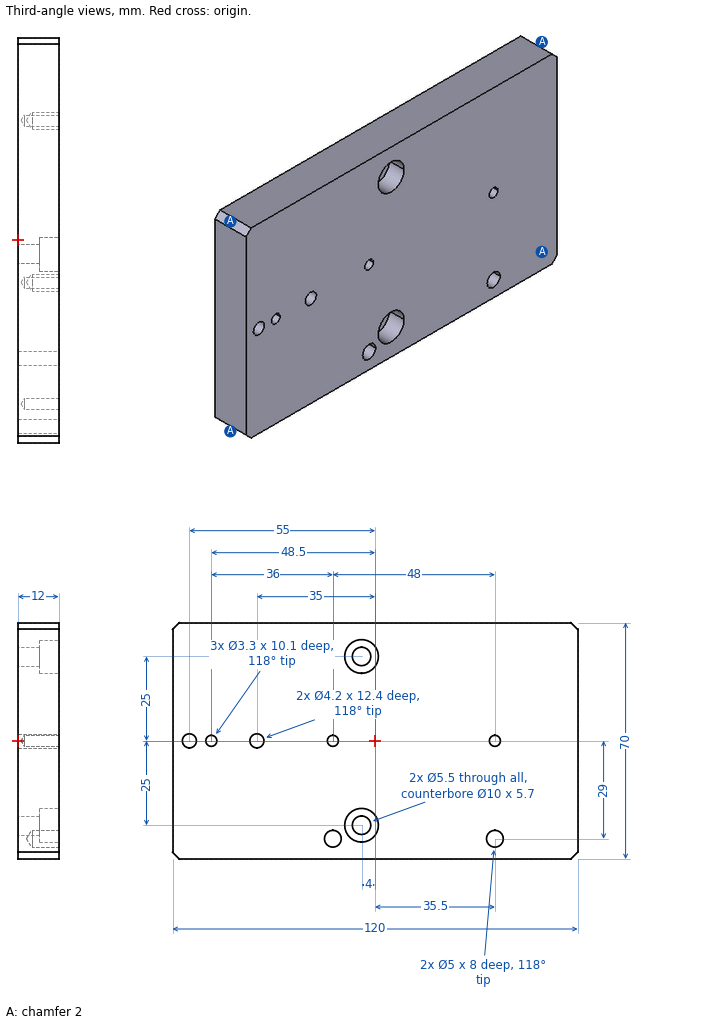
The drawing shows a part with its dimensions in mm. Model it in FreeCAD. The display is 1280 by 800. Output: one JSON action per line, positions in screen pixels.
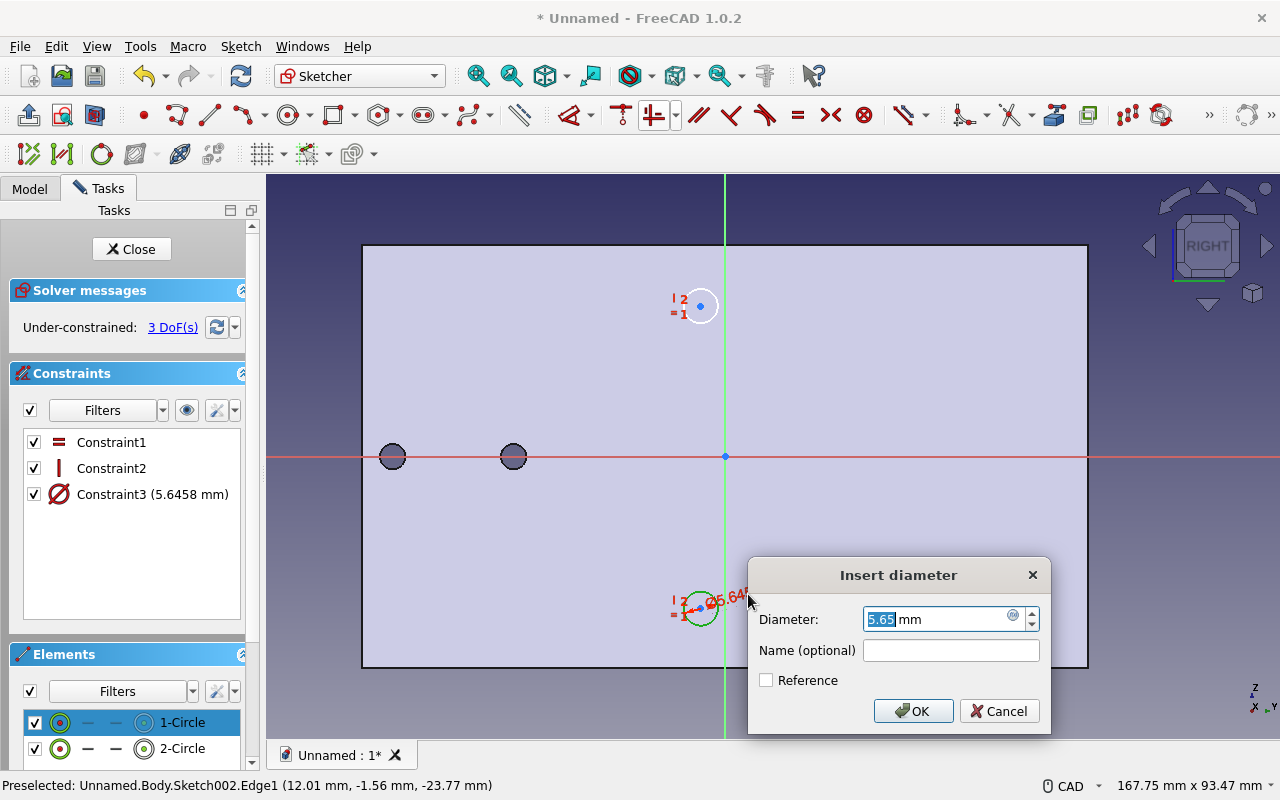
{"action": "type", "text": "5.5"}
{"action": "key", "text": "Return"}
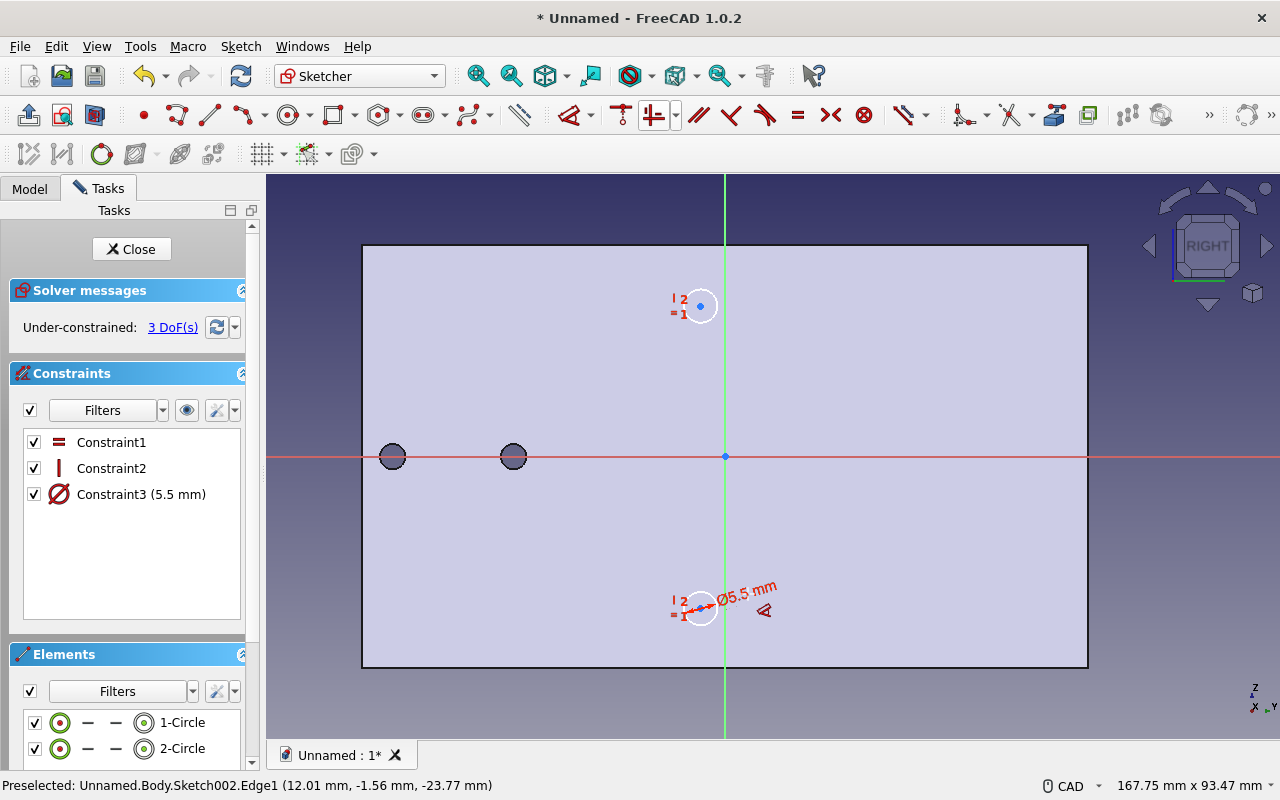
{"action": "scroll", "coordinate": [701, 609], "scroll_direction": "up", "scroll_amount": 3}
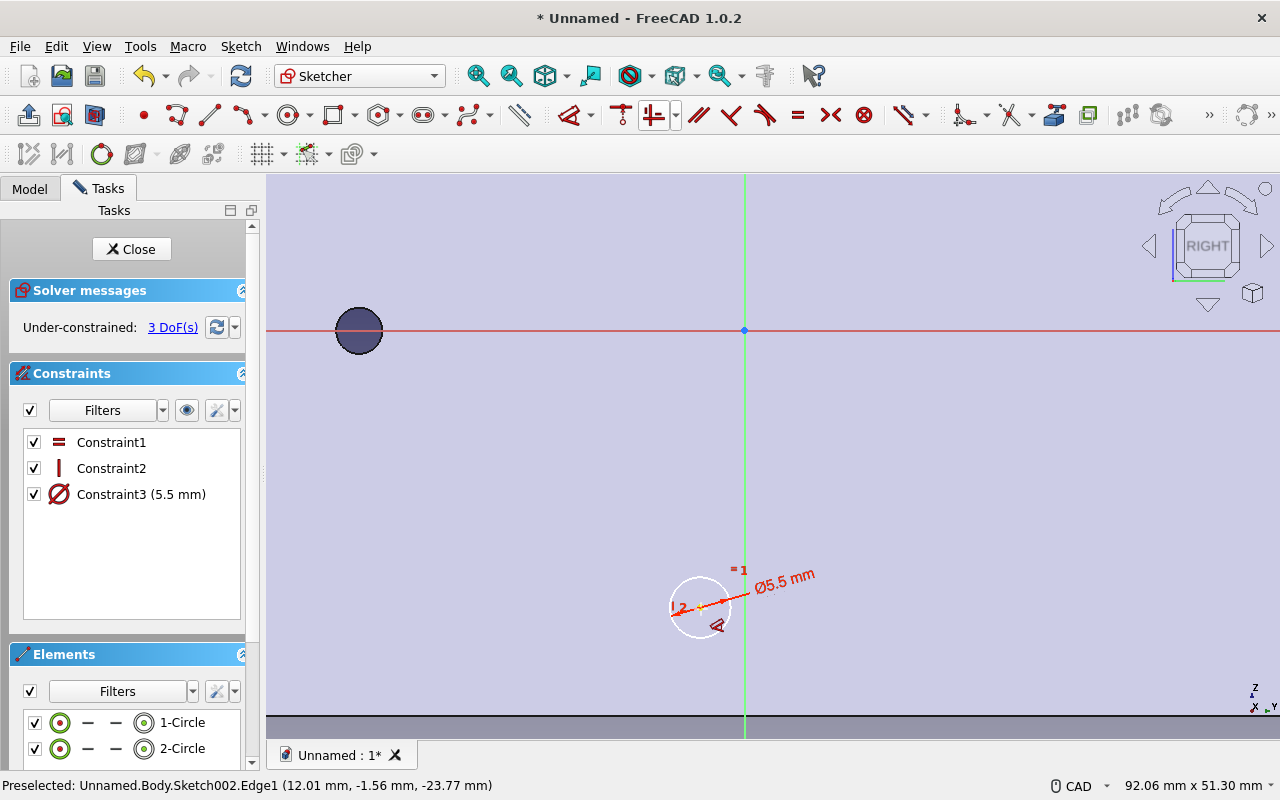
{"action": "left_click", "coordinate": [700, 608]}
{"action": "left_click", "coordinate": [722, 297]}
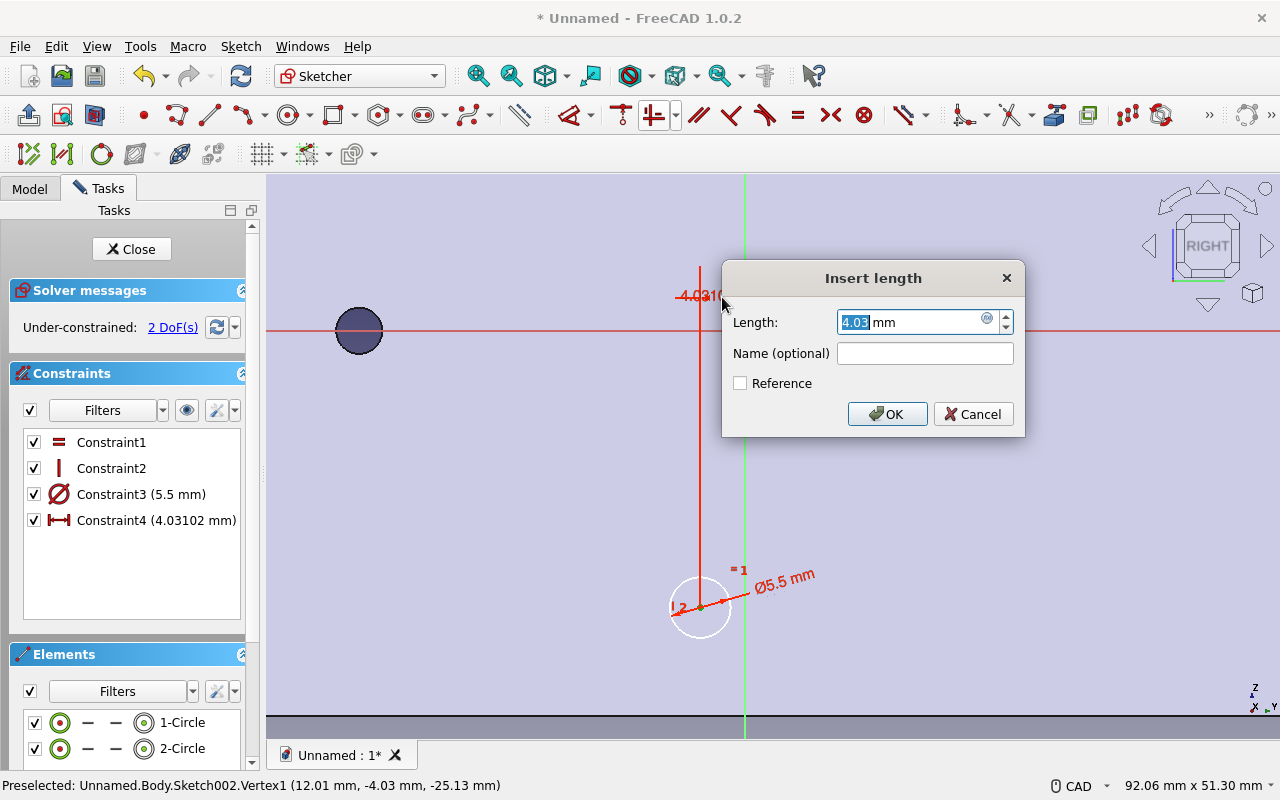
{"action": "type", "text": "4"}
{"action": "key", "text": "Return"}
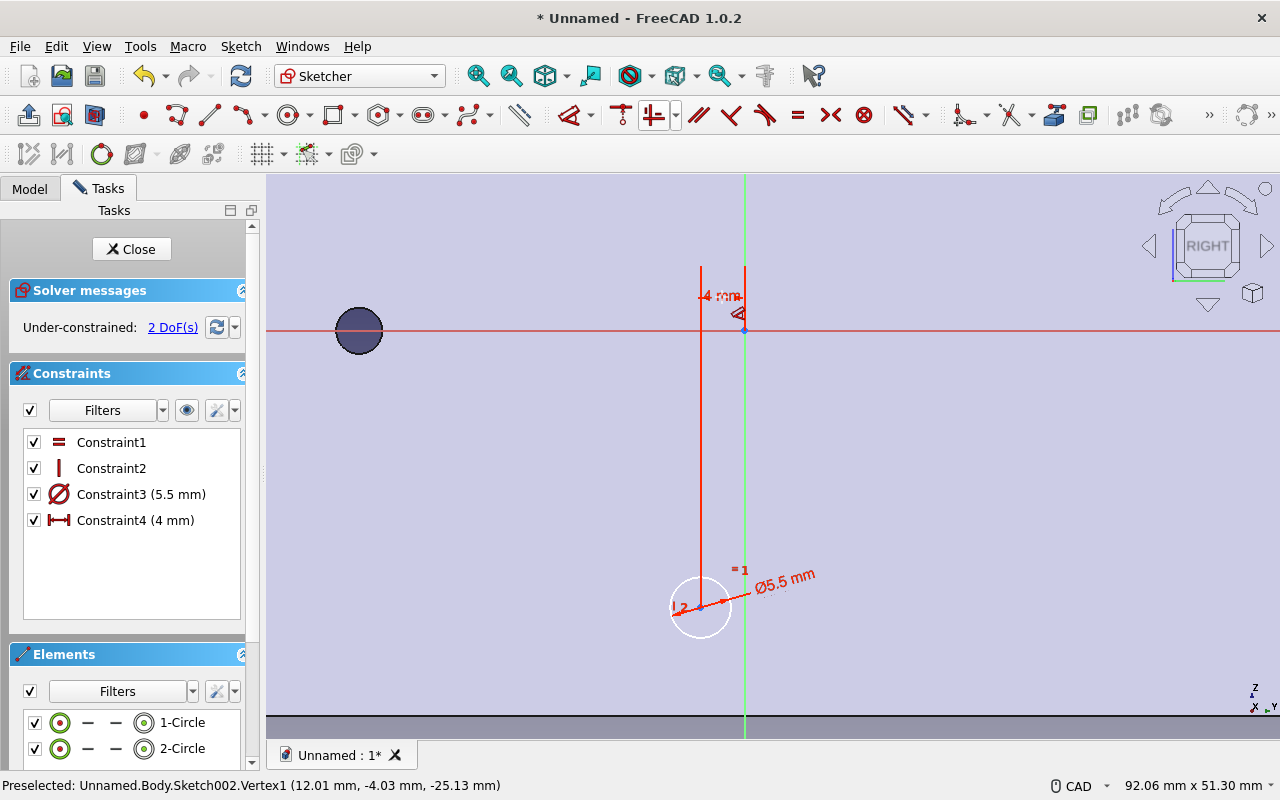
{"action": "left_click", "coordinate": [701, 608]}
{"action": "left_click", "coordinate": [779, 469]}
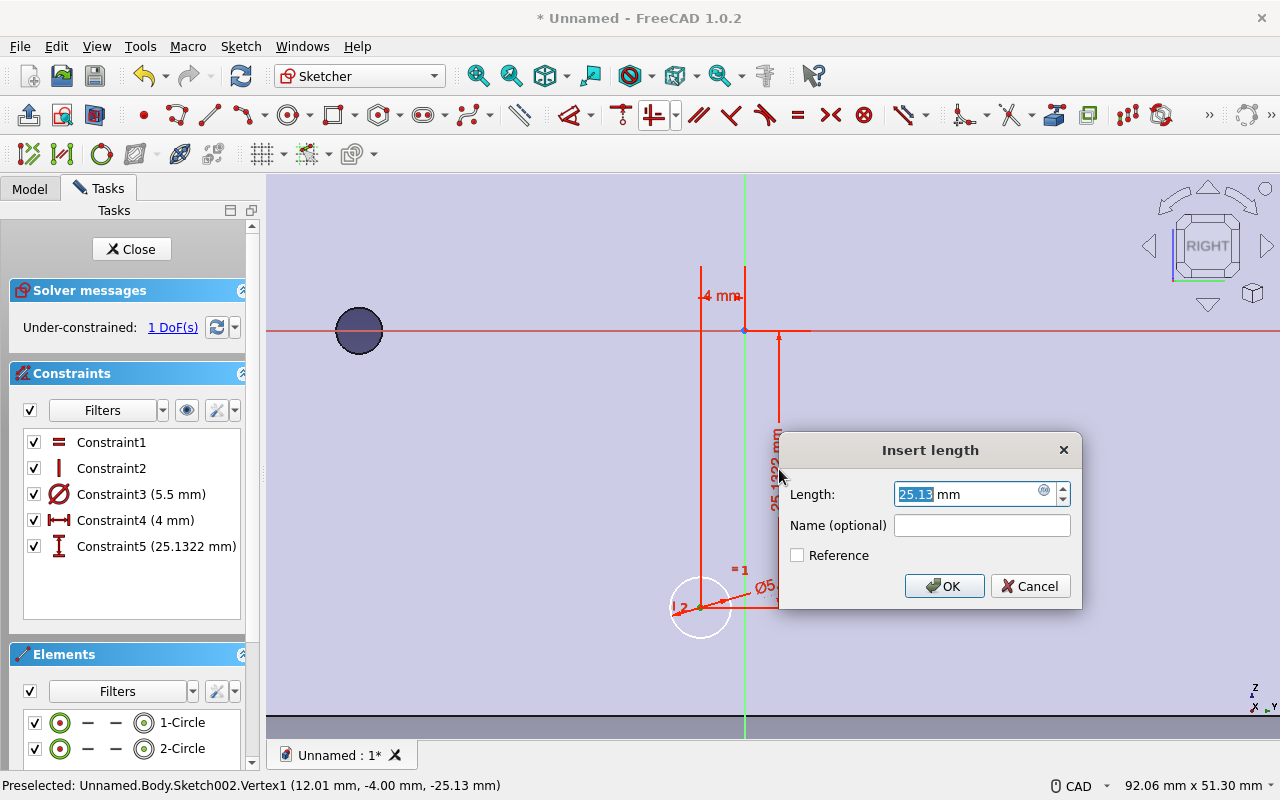
{"action": "type", "text": "25"}
{"action": "key", "text": "Return"}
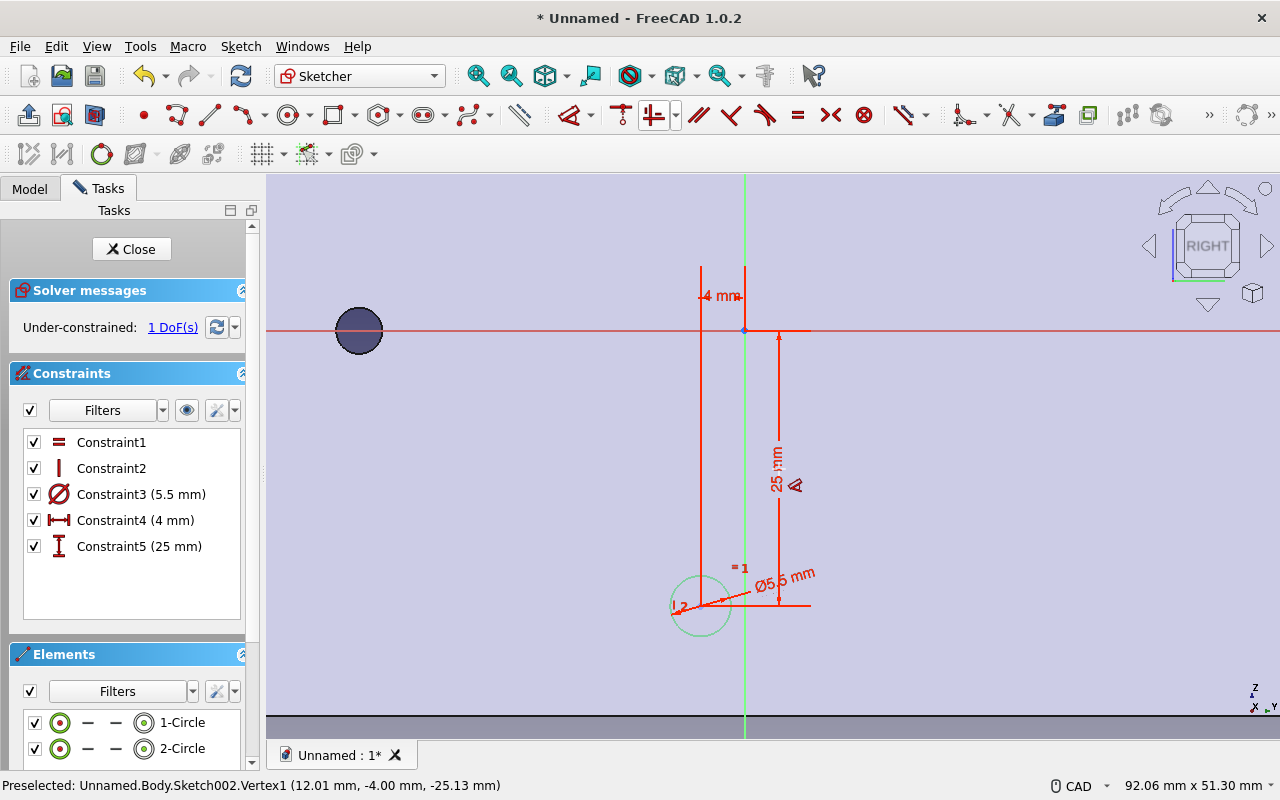
{"action": "scroll", "coordinate": [701, 609], "scroll_direction": "down", "scroll_amount": 3}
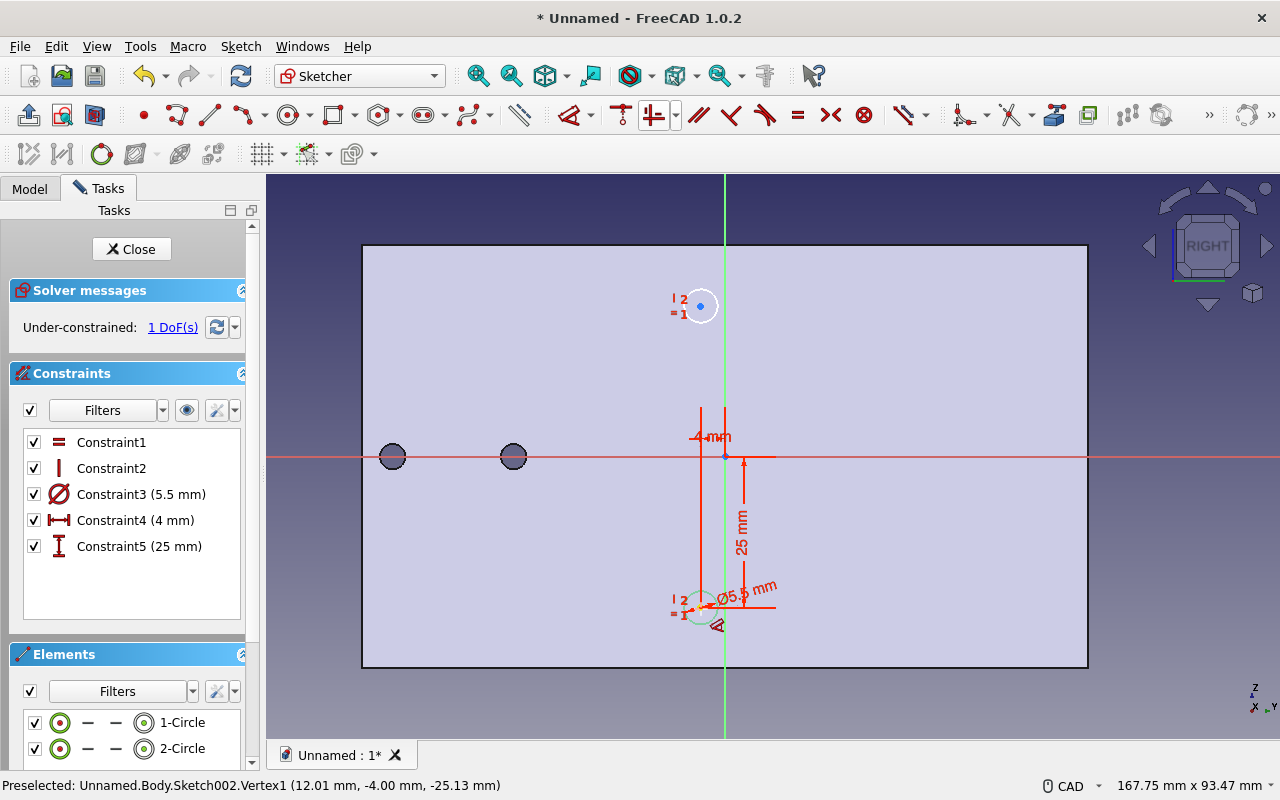
{"action": "left_click", "coordinate": [701, 306]}
{"action": "left_click", "coordinate": [759, 381]}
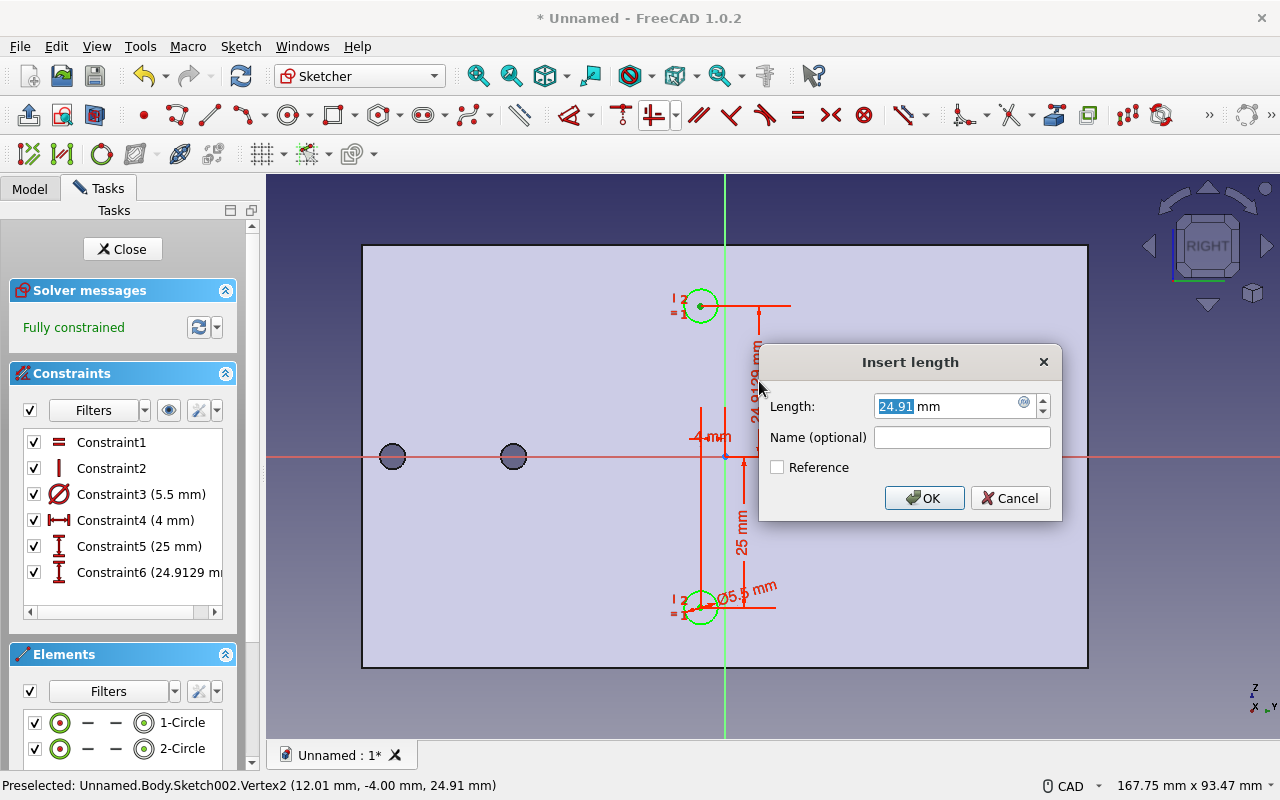
{"action": "type", "text": "25"}
{"action": "key", "text": "Return"}
{"action": "key", "text": "Escape"}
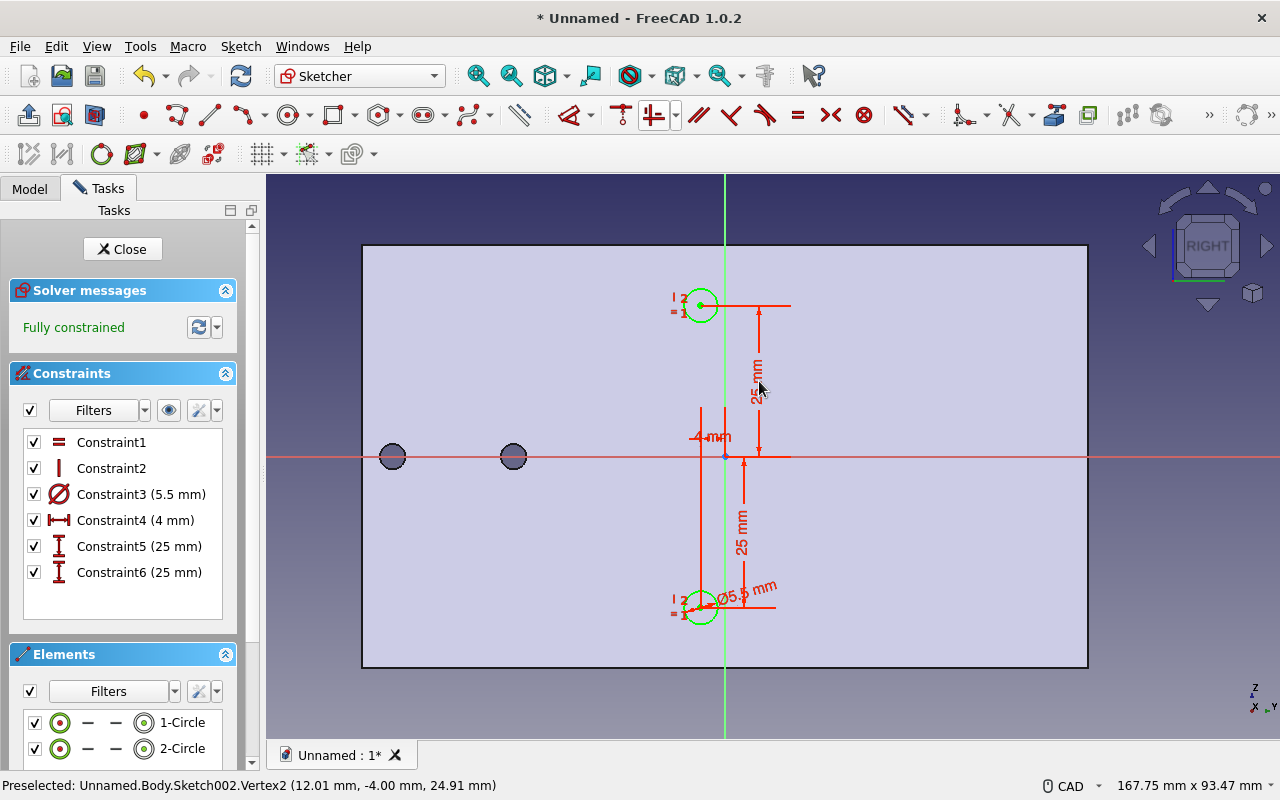
{"action": "left_click", "coordinate": [123, 249]}